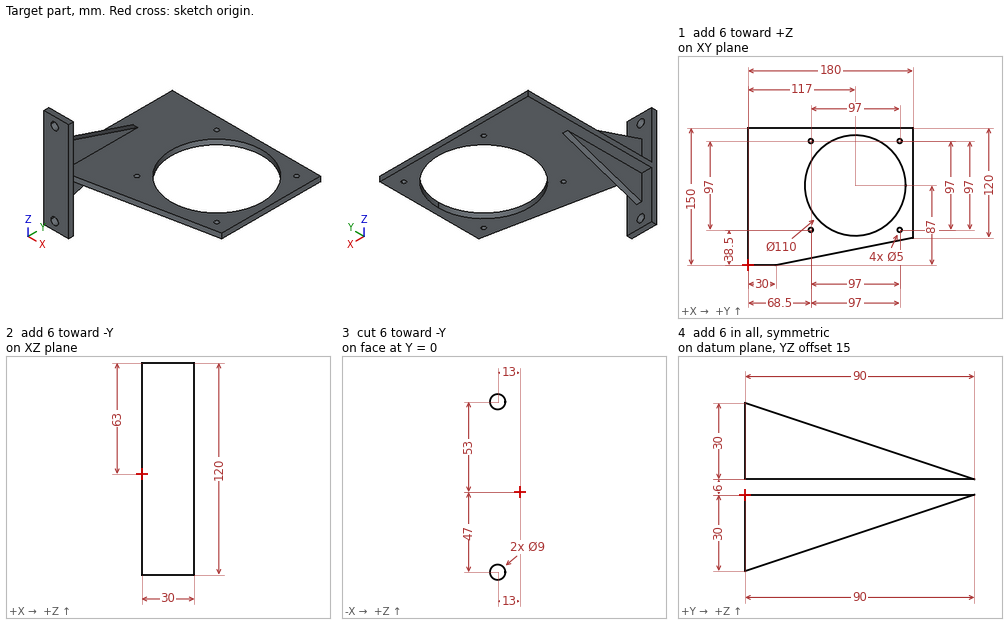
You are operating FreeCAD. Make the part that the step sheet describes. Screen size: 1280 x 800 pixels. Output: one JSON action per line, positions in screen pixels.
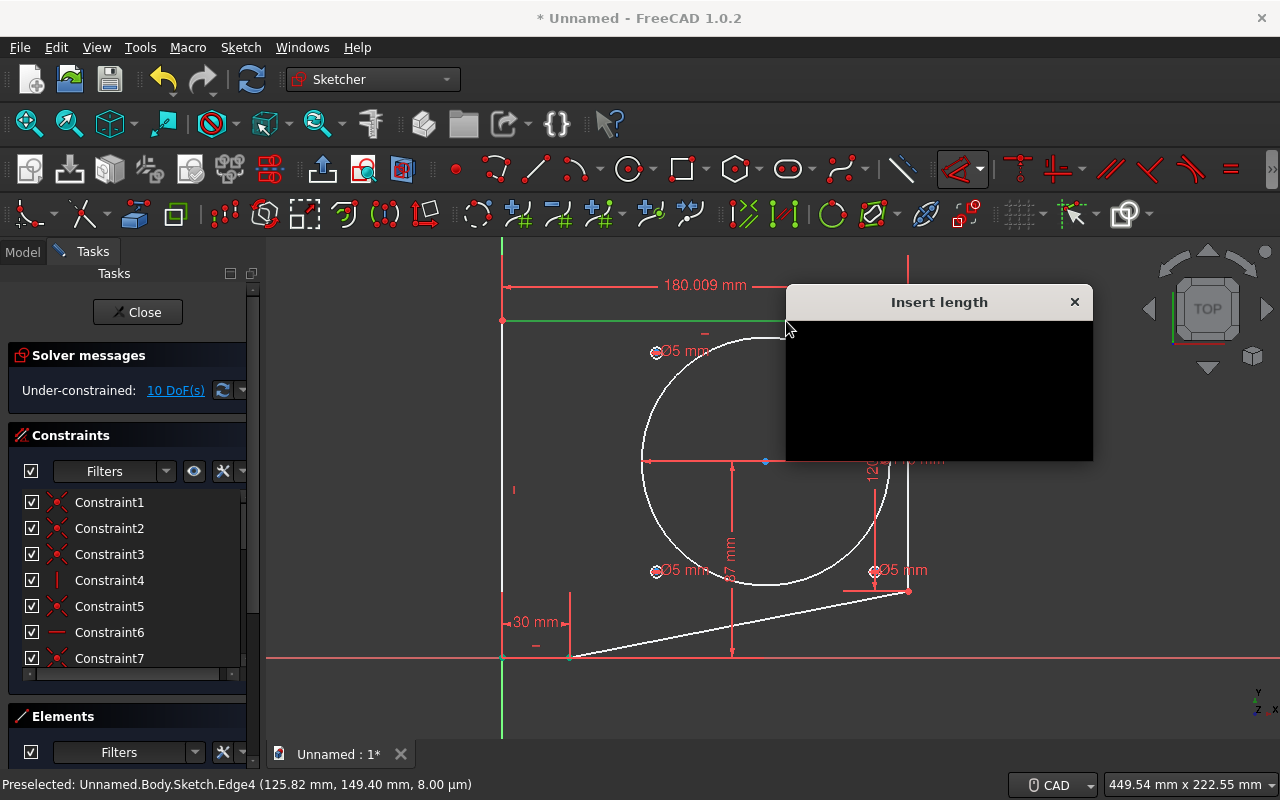
{"action": "type", "text": "180"}
{"action": "key", "text": "Return"}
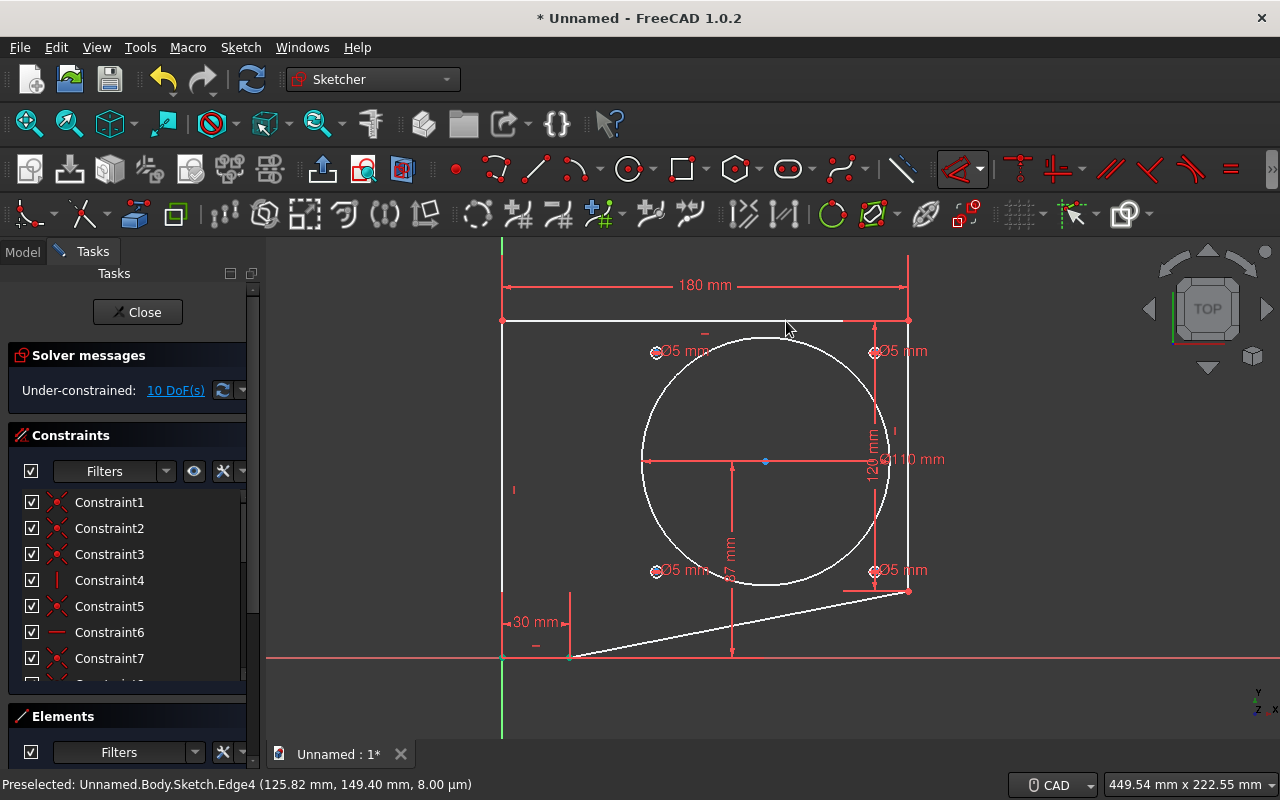
{"action": "left_click", "coordinate": [502, 422]}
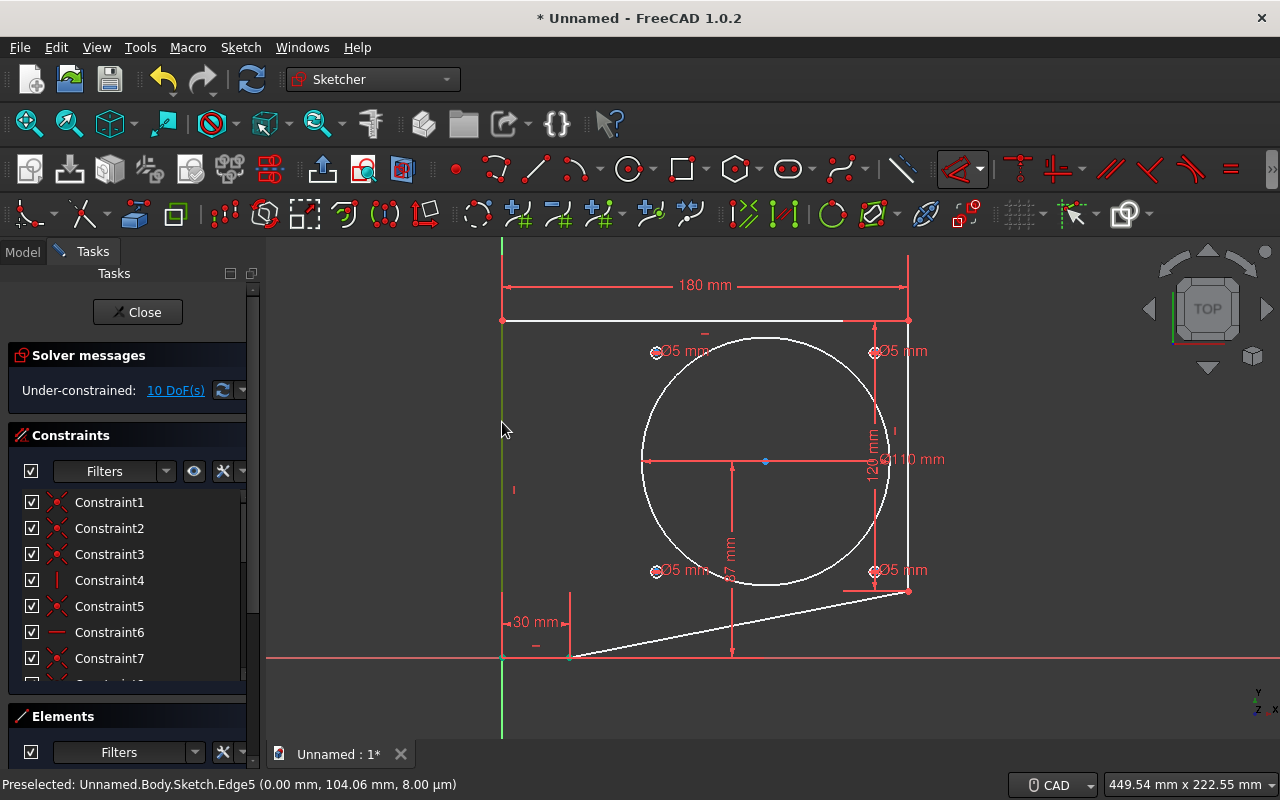
{"action": "key", "text": "i"}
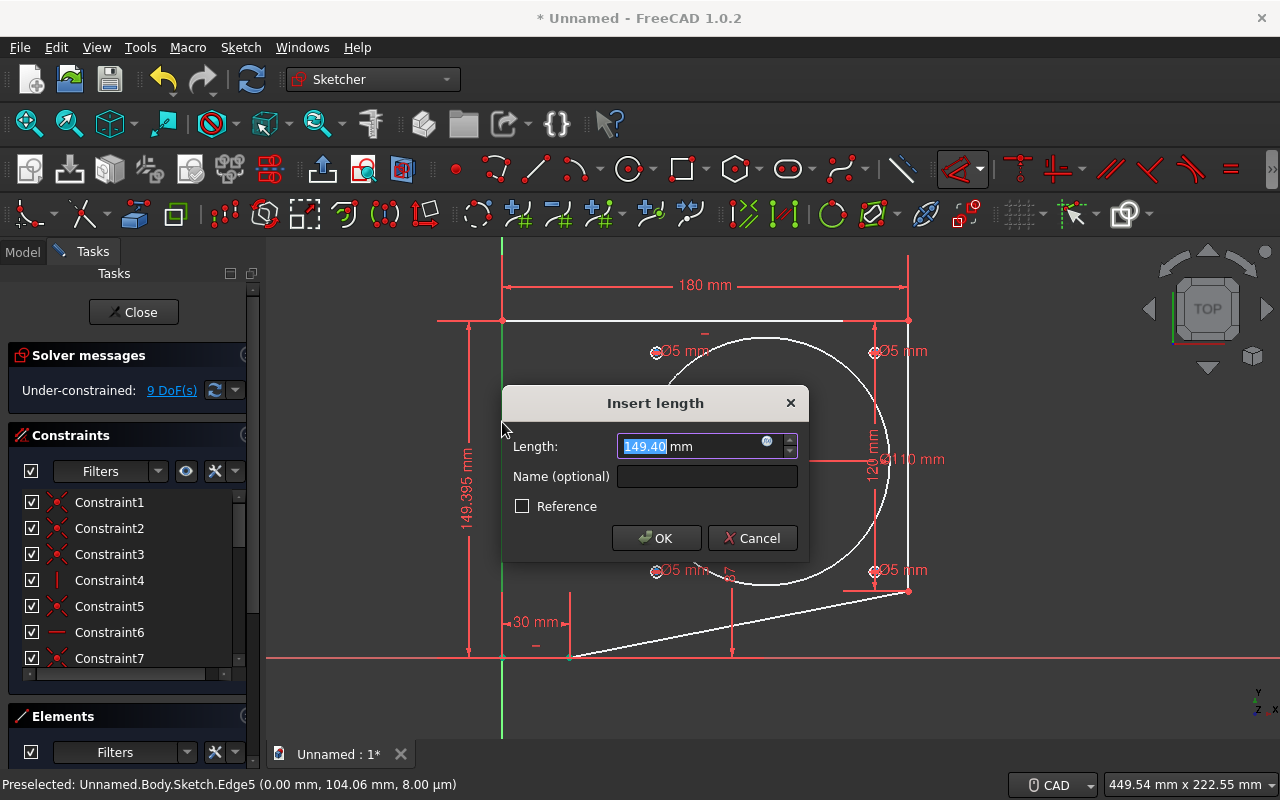
{"action": "type", "text": "150"}
{"action": "key", "text": "Return"}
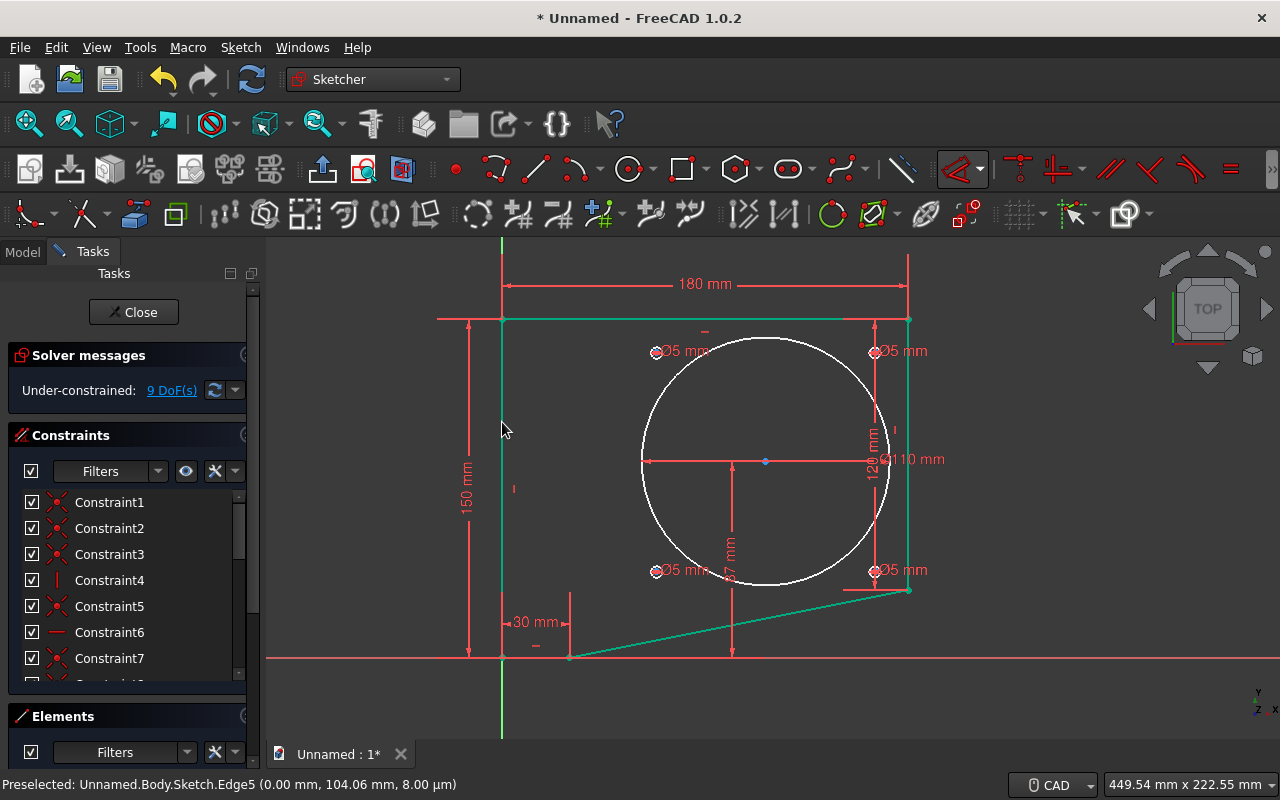
{"action": "left_click", "coordinate": [766, 461]}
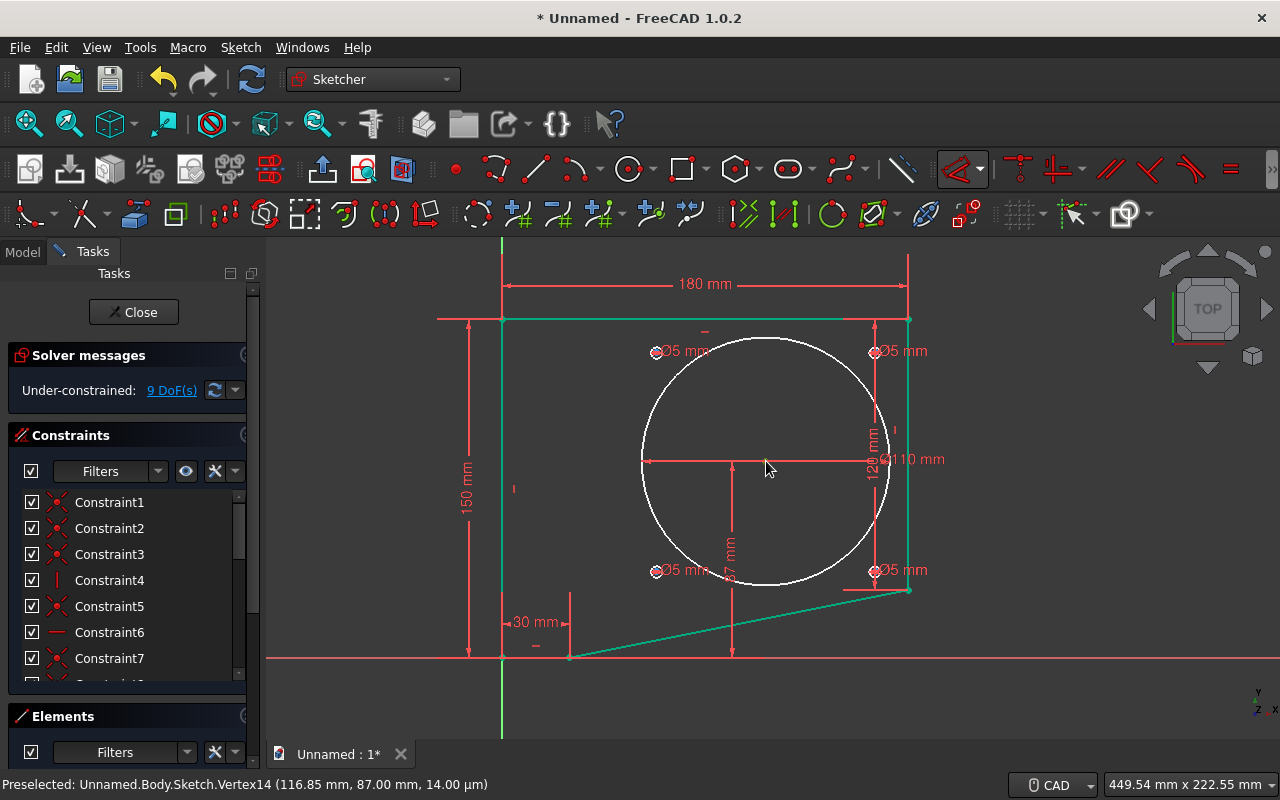
{"action": "key", "text": "l"}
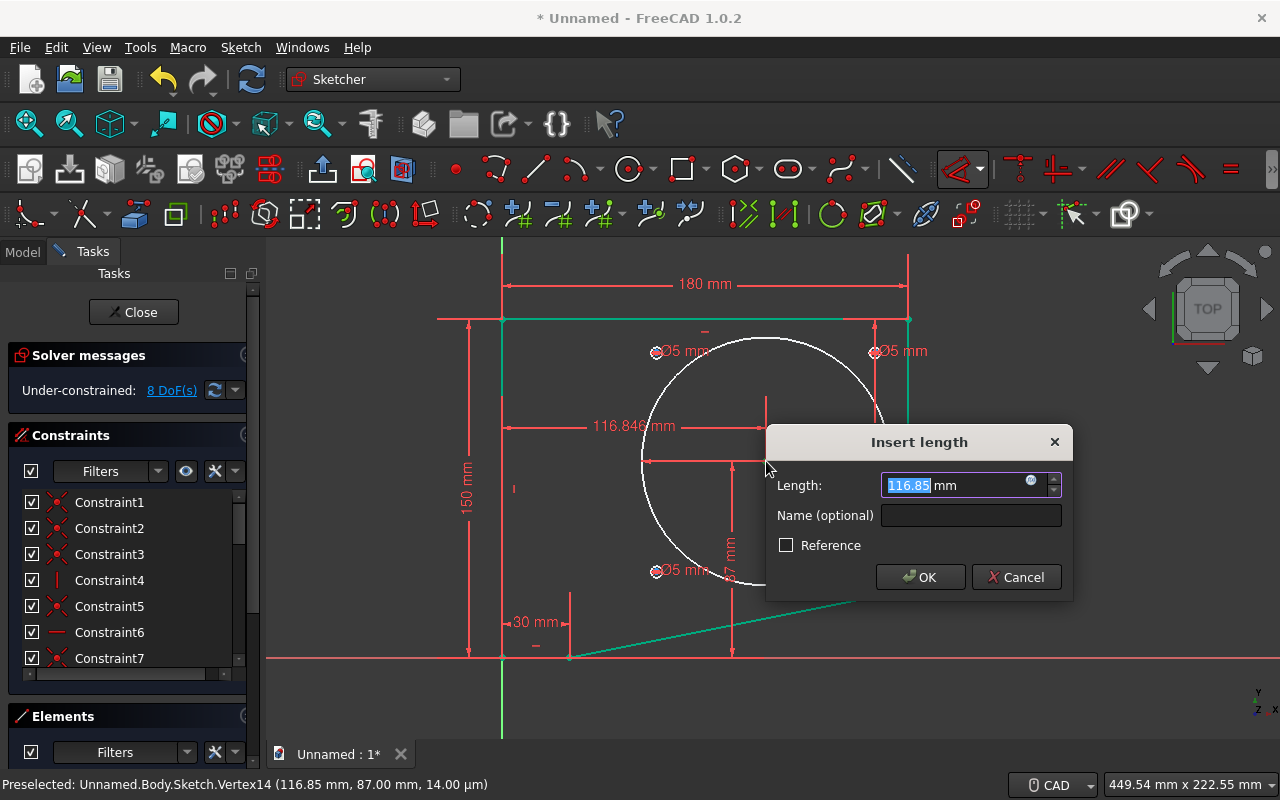
{"action": "type", "text": "117"}
{"action": "key", "text": "Return"}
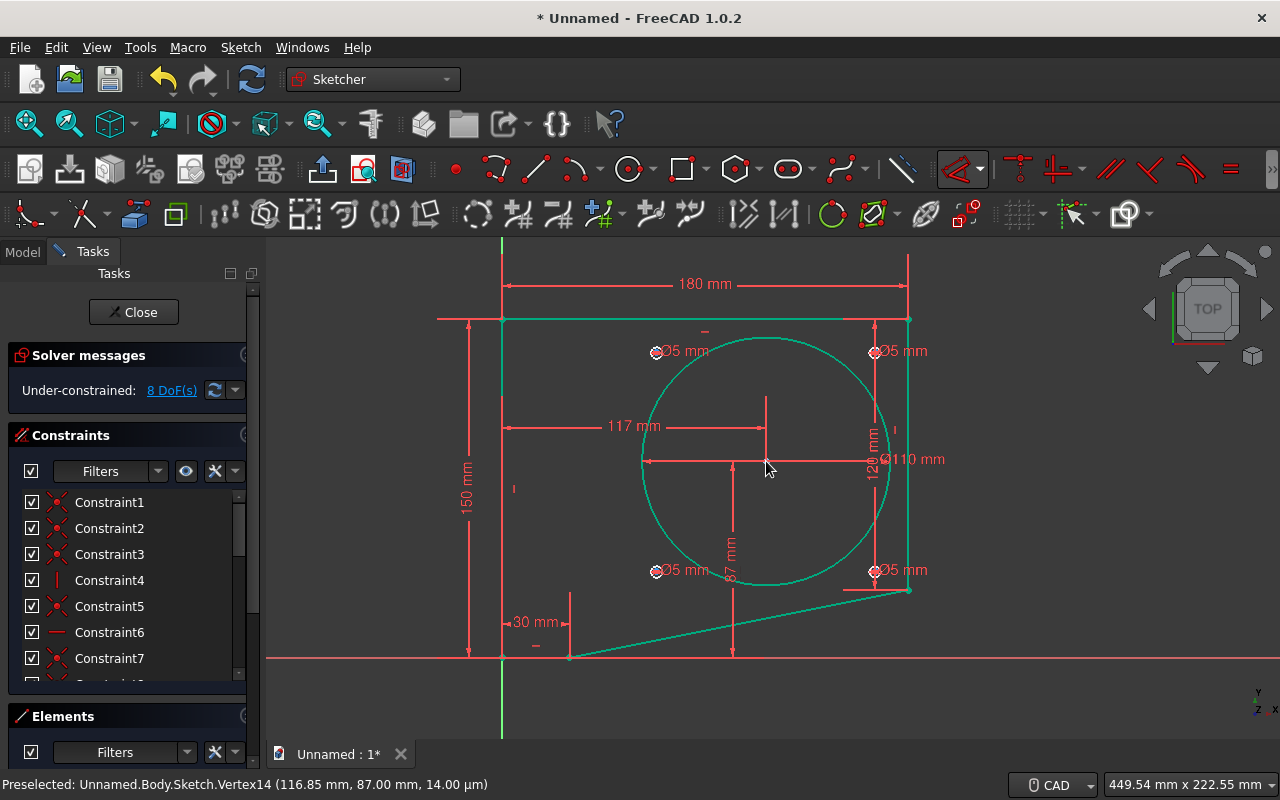
{"action": "left_click", "coordinate": [657, 572]}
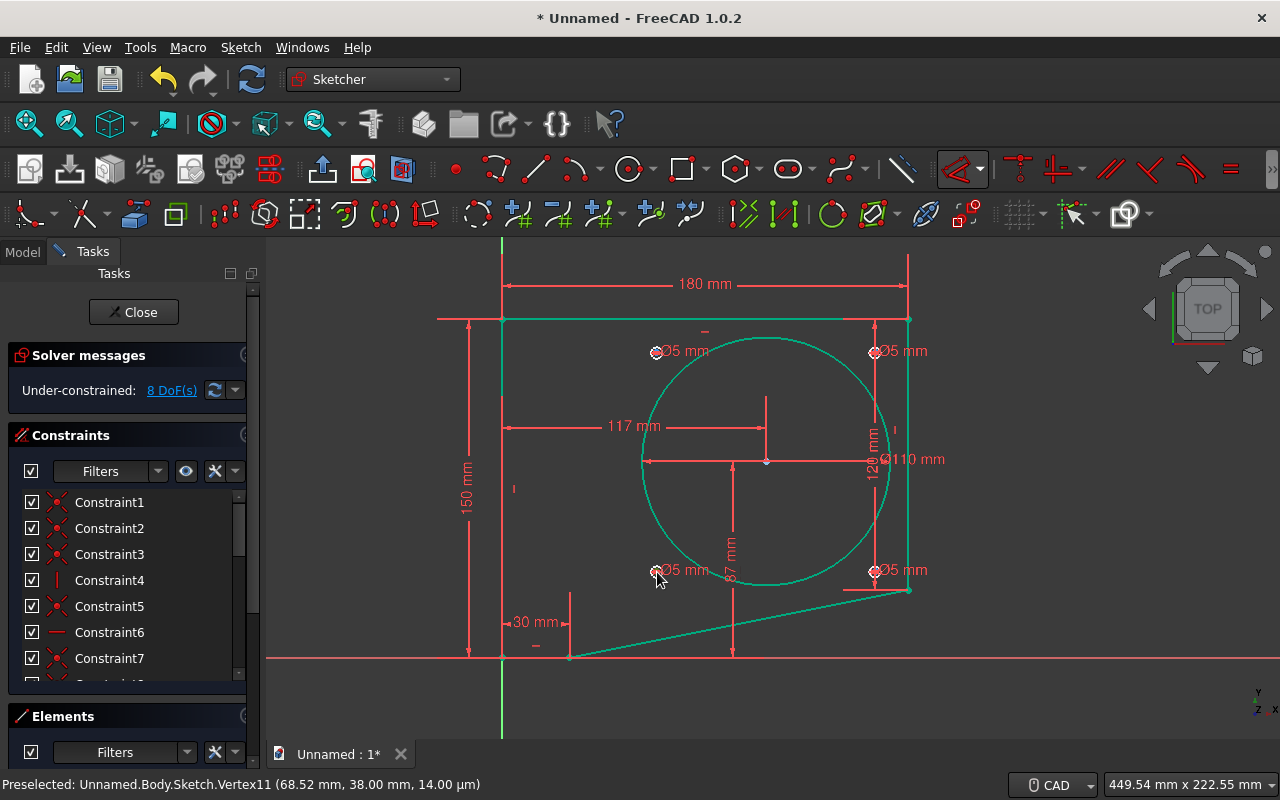
{"action": "left_click", "coordinate": [875, 572]}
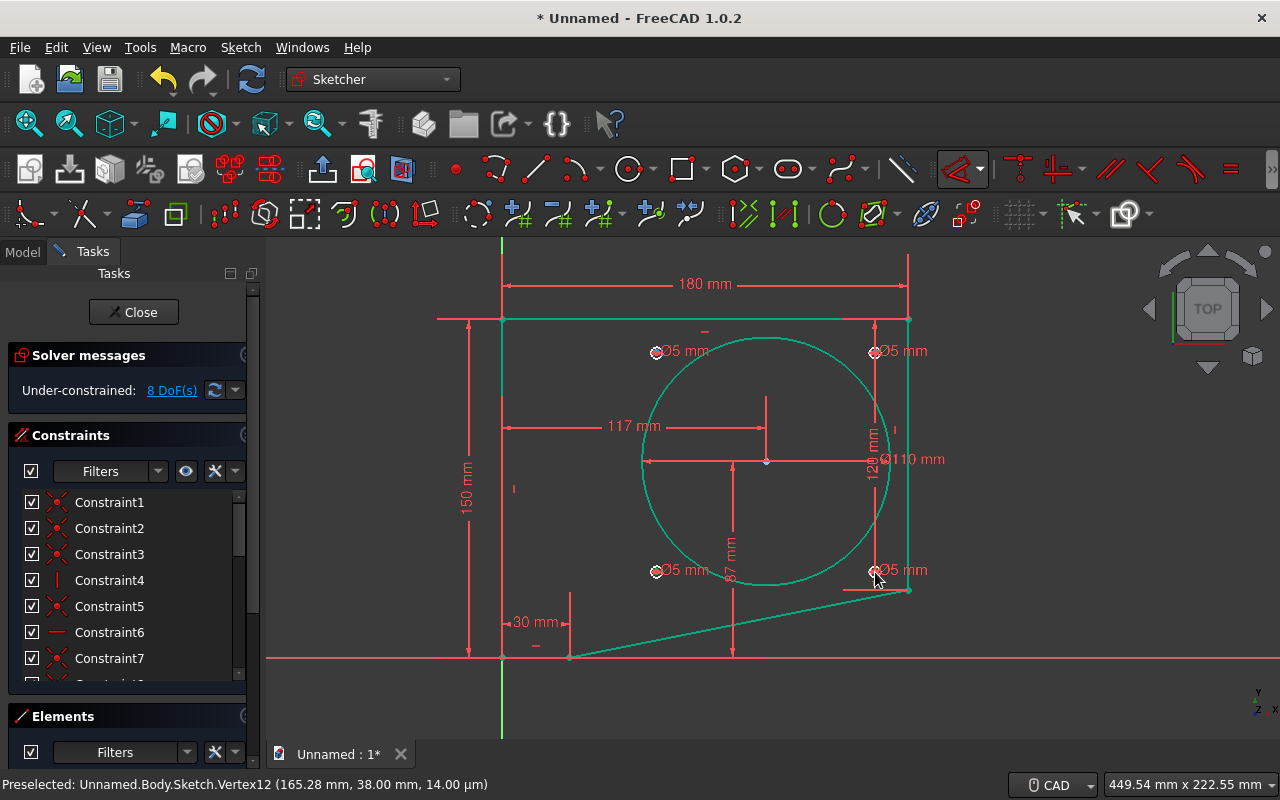
{"action": "key", "text": "l"}